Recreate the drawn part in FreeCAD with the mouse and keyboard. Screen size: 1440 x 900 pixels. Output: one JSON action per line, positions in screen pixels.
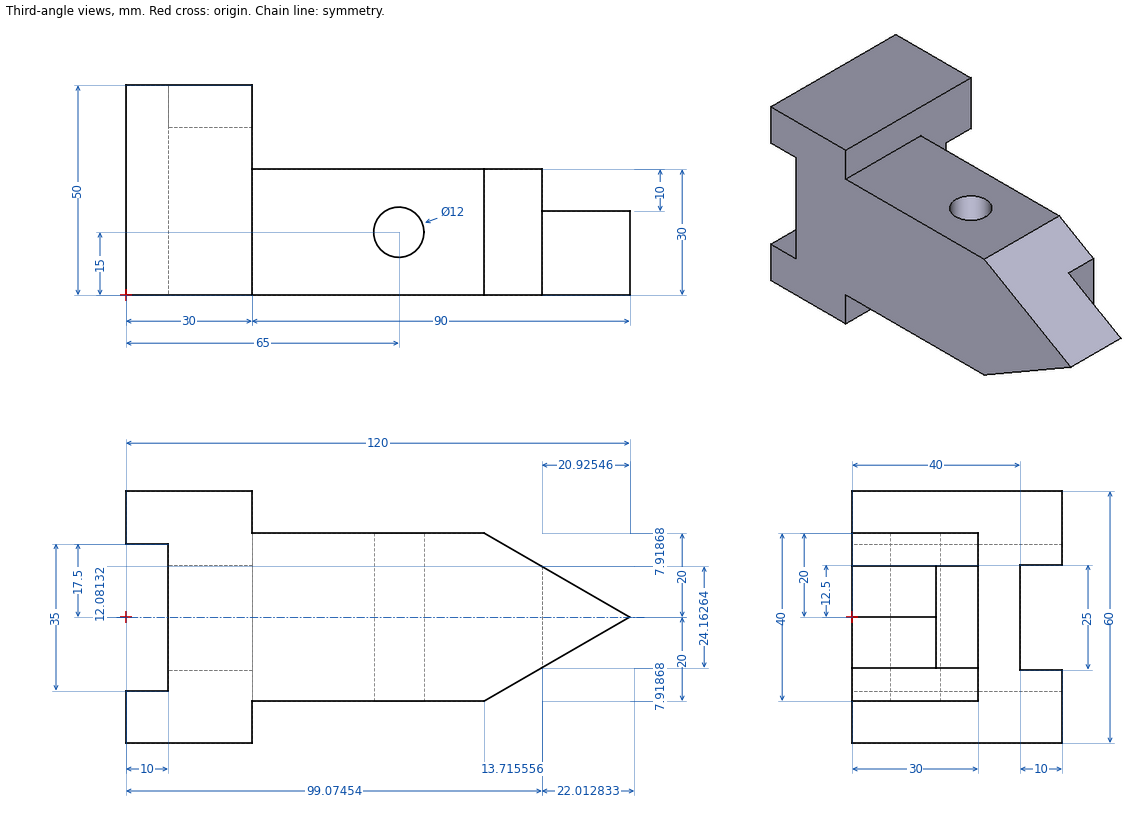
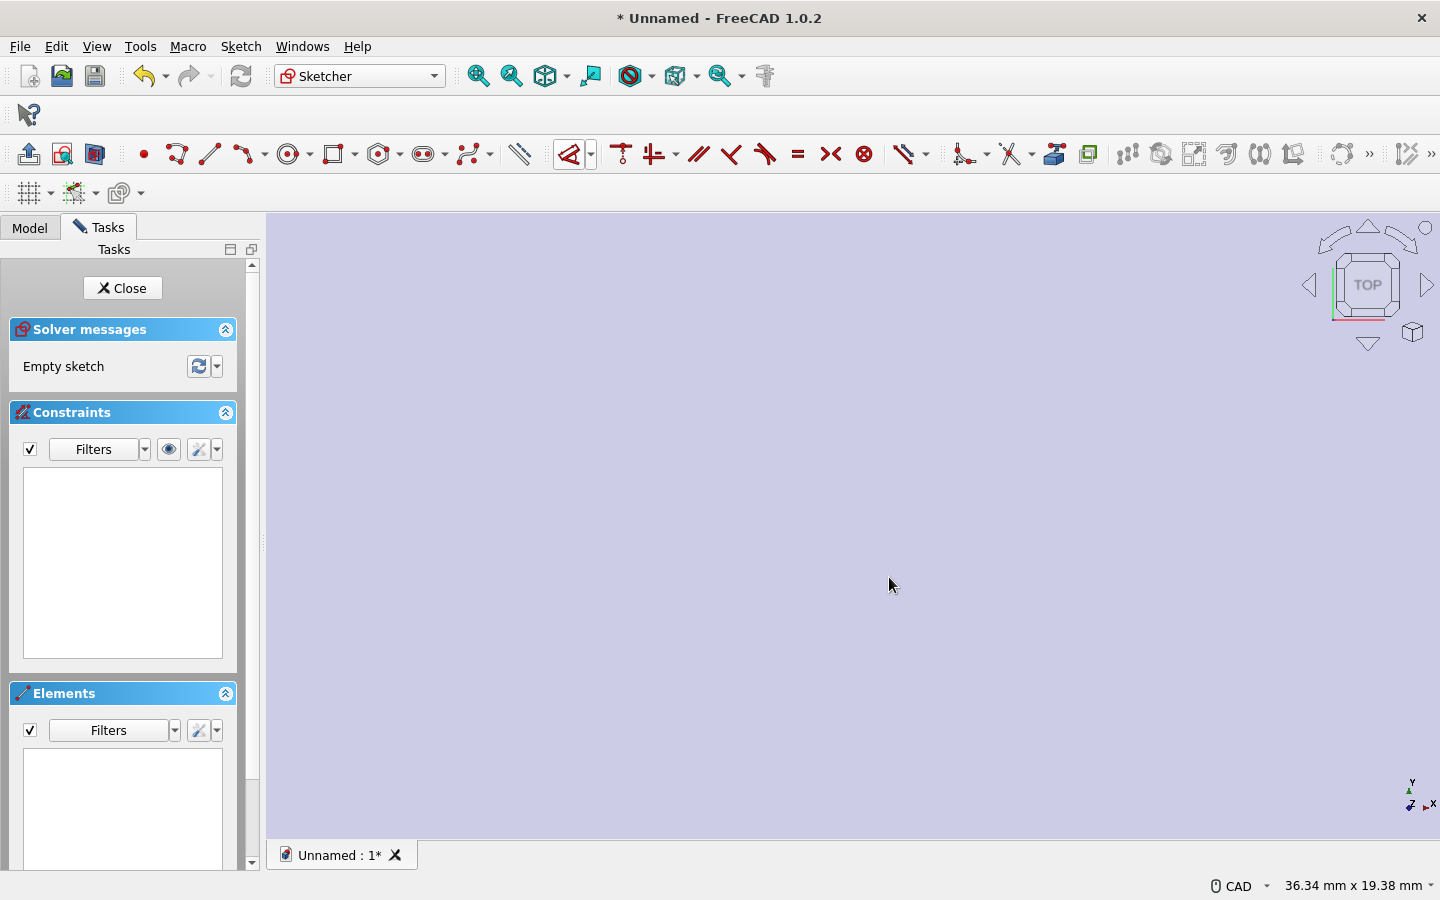
{"action": "left_click", "coordinate": [288, 154]}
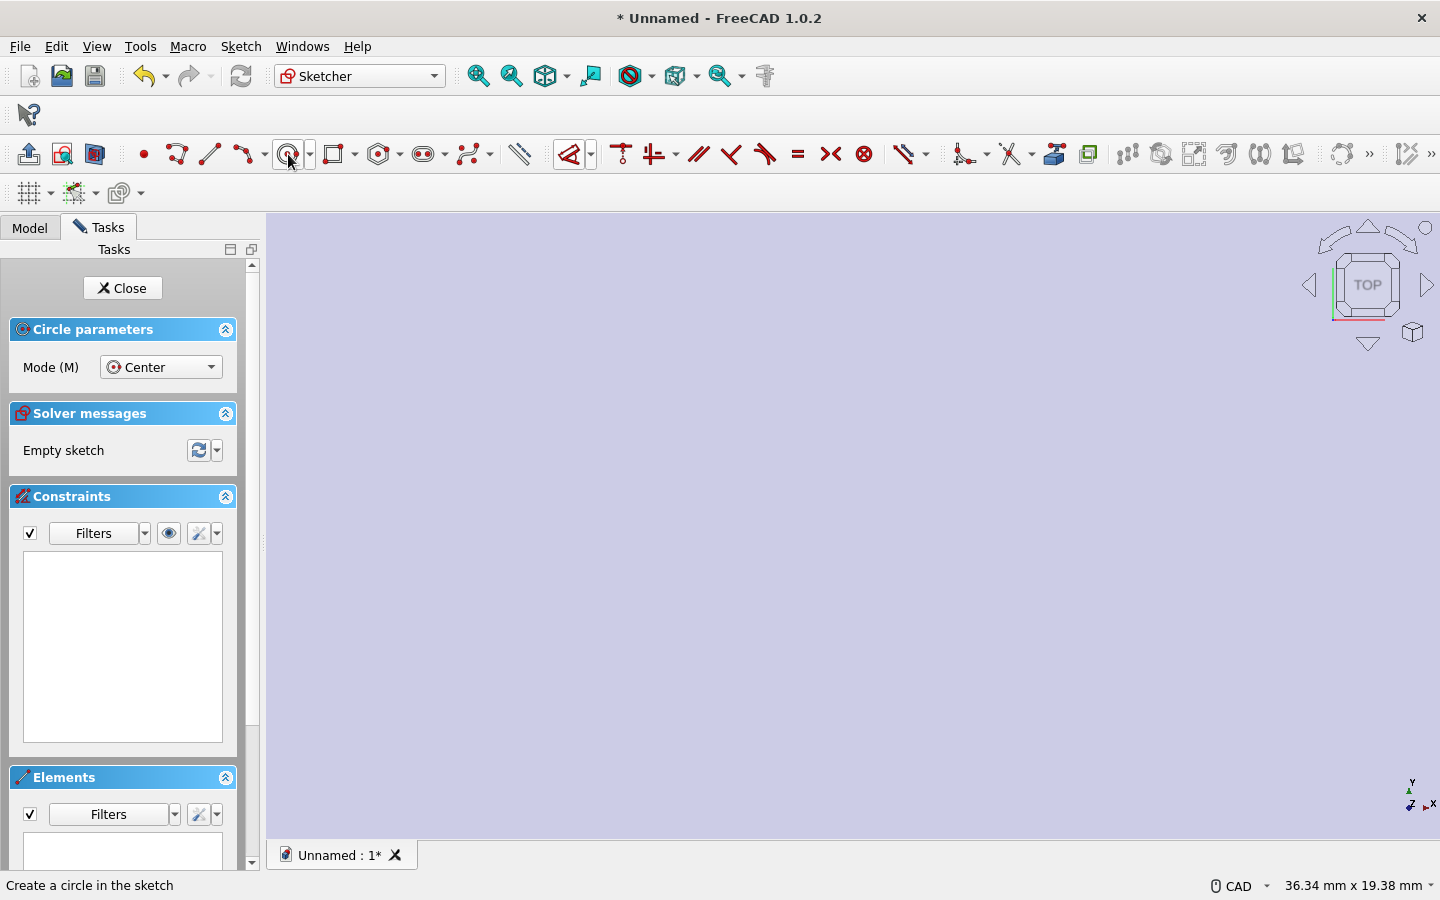
{"action": "left_click", "coordinate": [781, 519]}
{"action": "left_click", "coordinate": [918, 382]}
{"action": "key", "text": "Escape"}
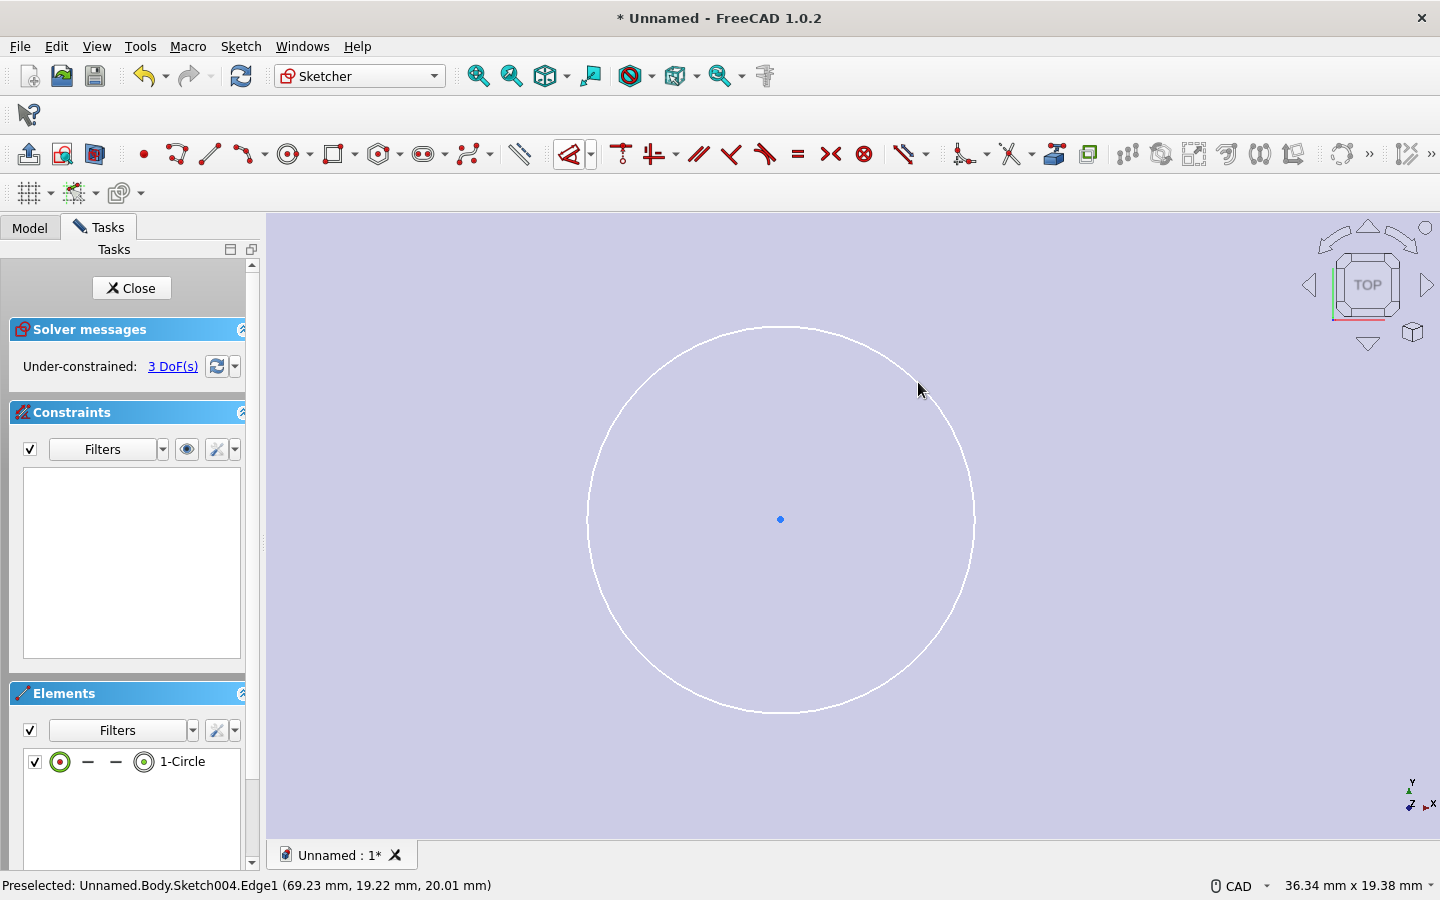
{"action": "left_click", "coordinate": [918, 383]}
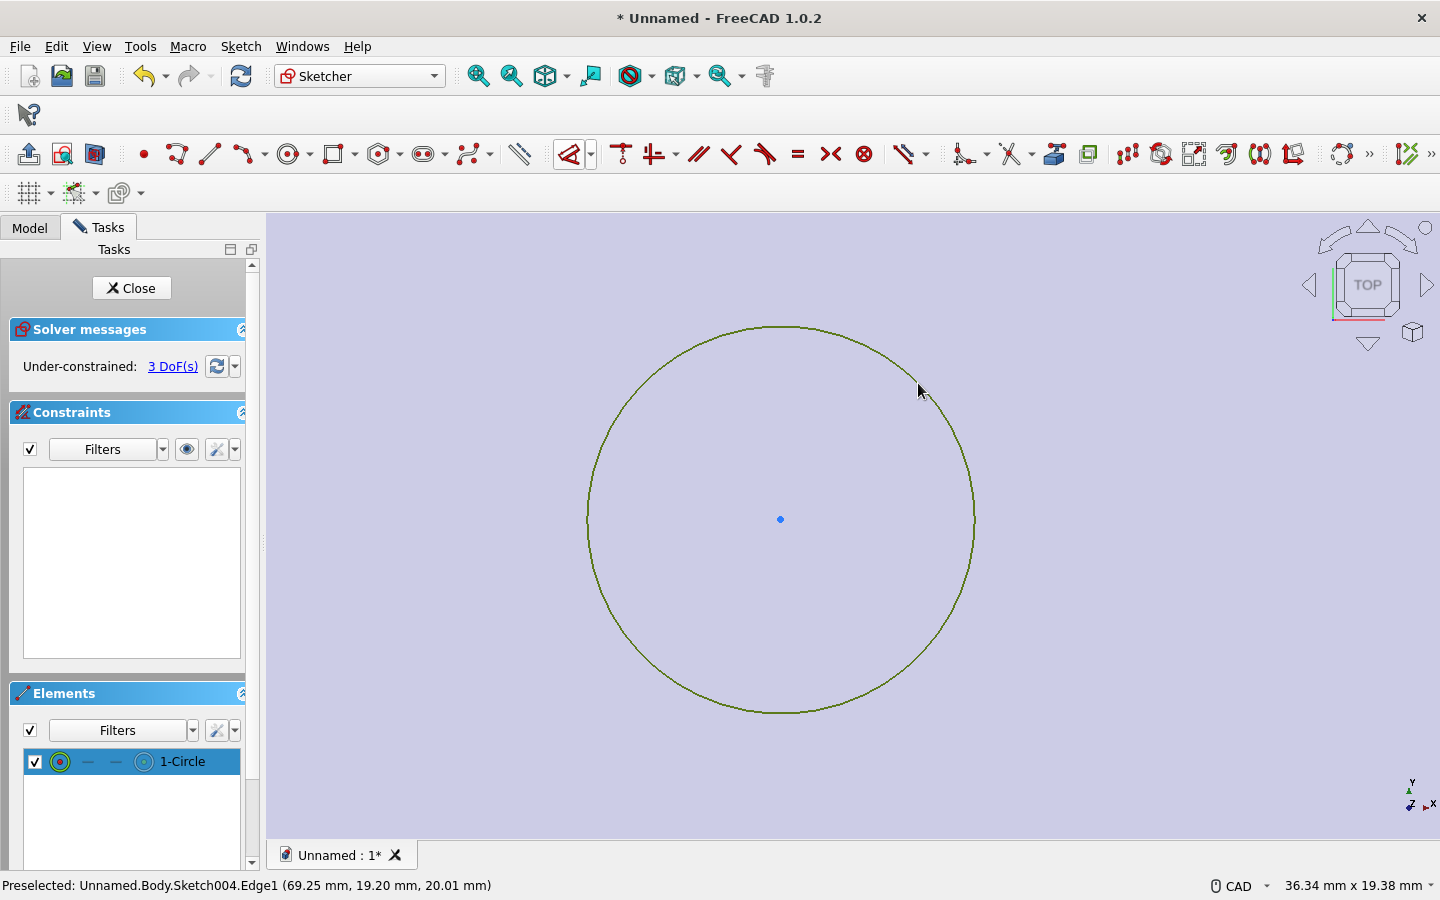
{"action": "left_click", "coordinate": [590, 154]}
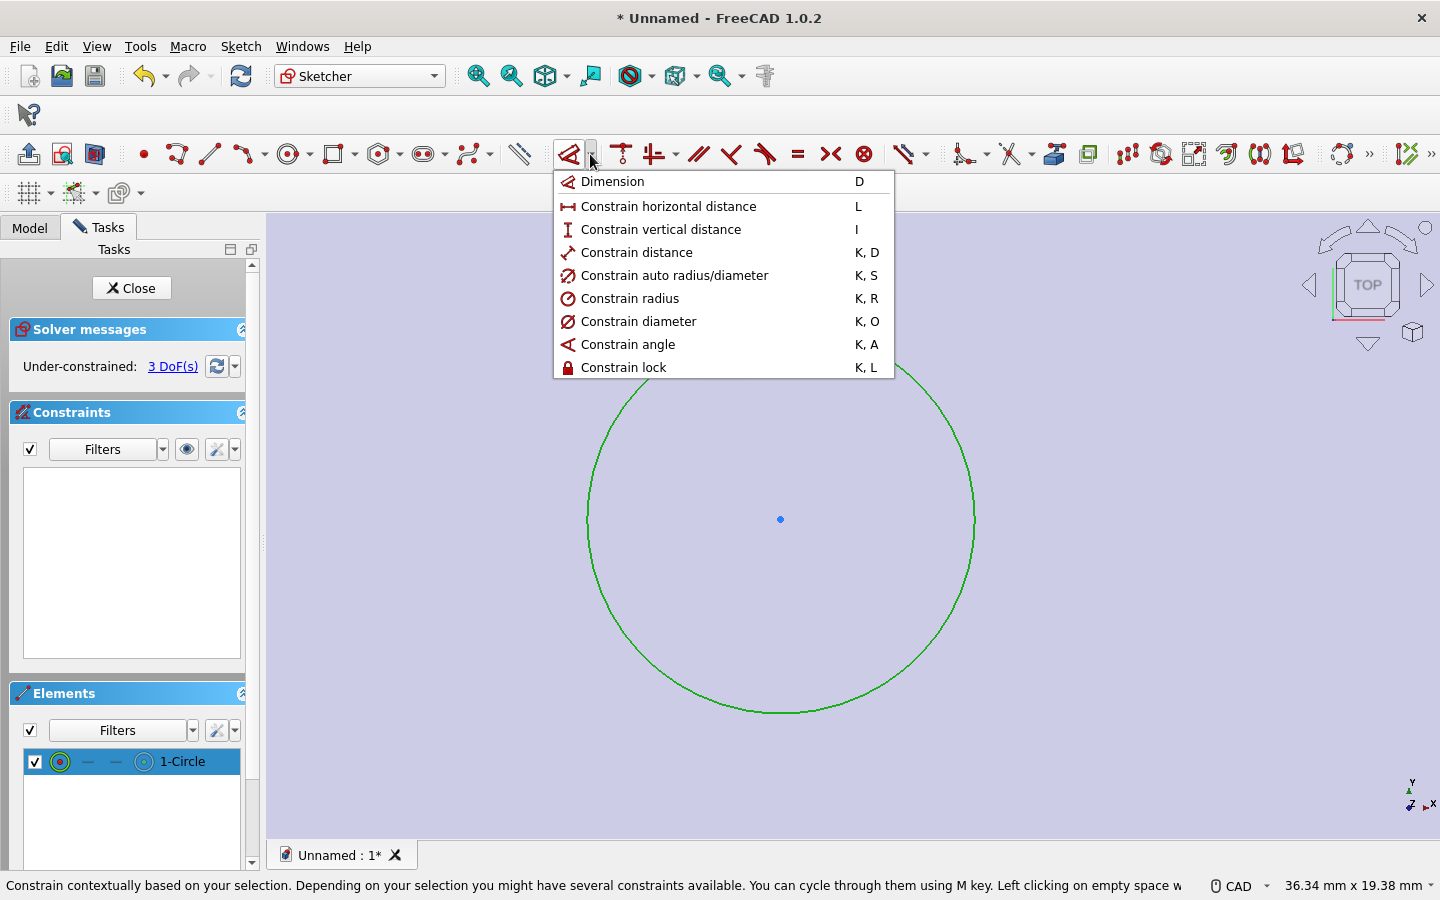
{"action": "left_click", "coordinate": [724, 322]}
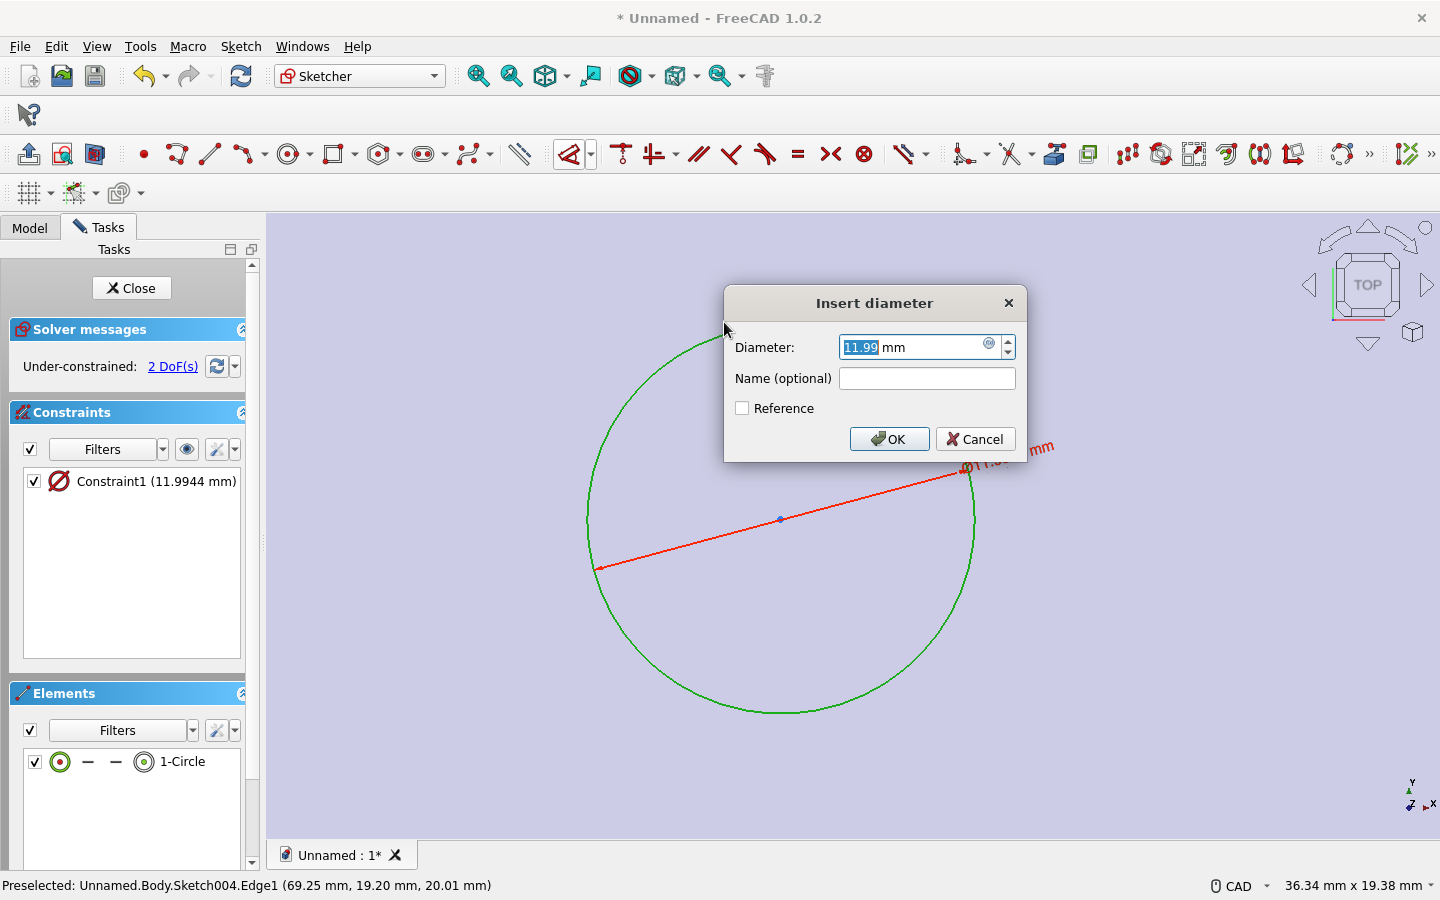
{"action": "type", "text": "12"}
{"action": "key", "text": "Return"}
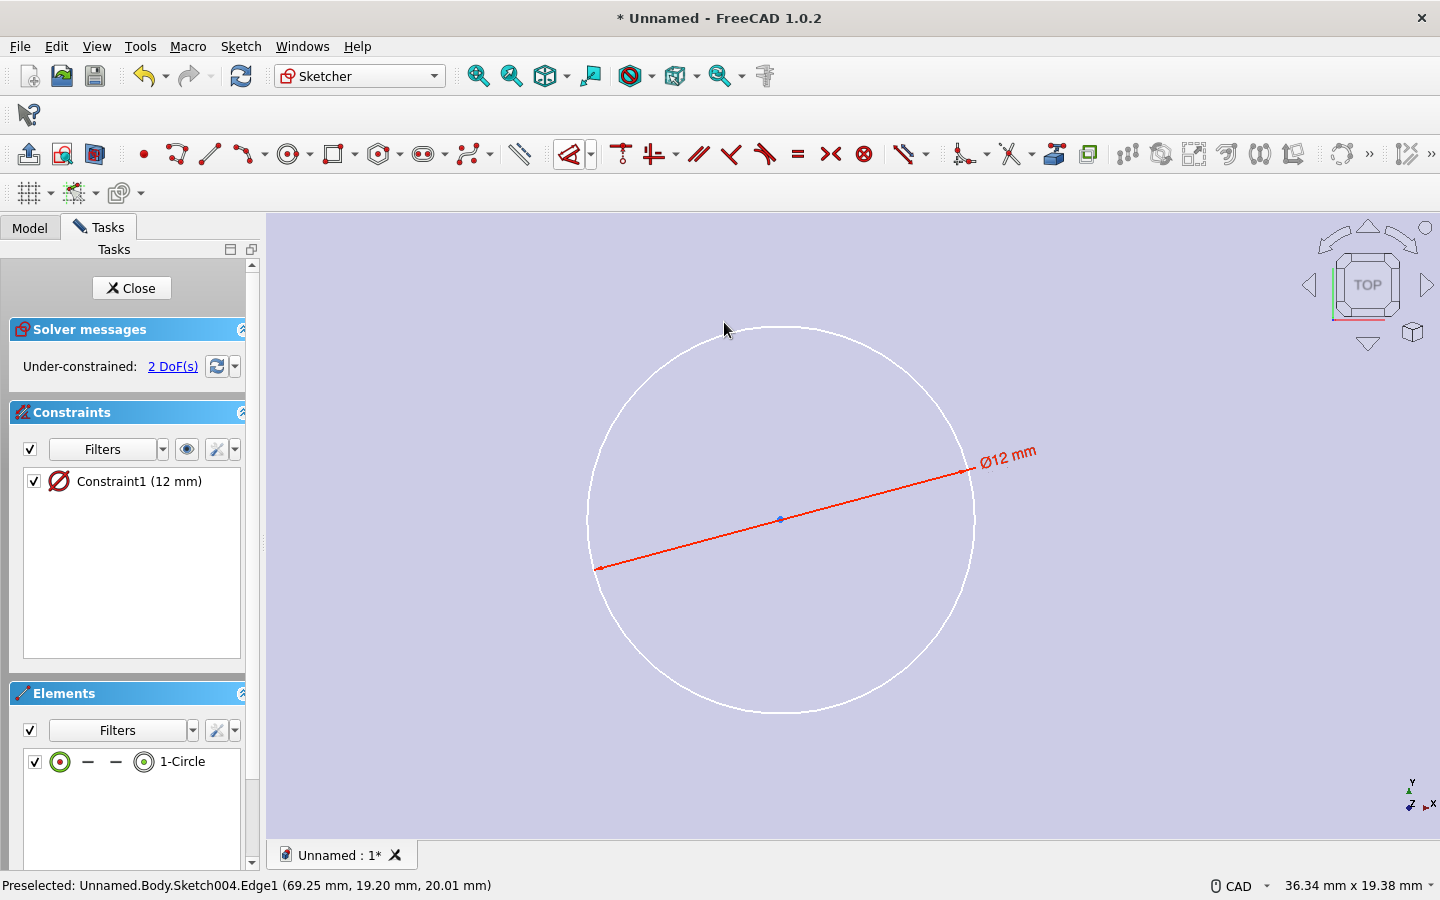
{"action": "left_click", "coordinate": [781, 520]}